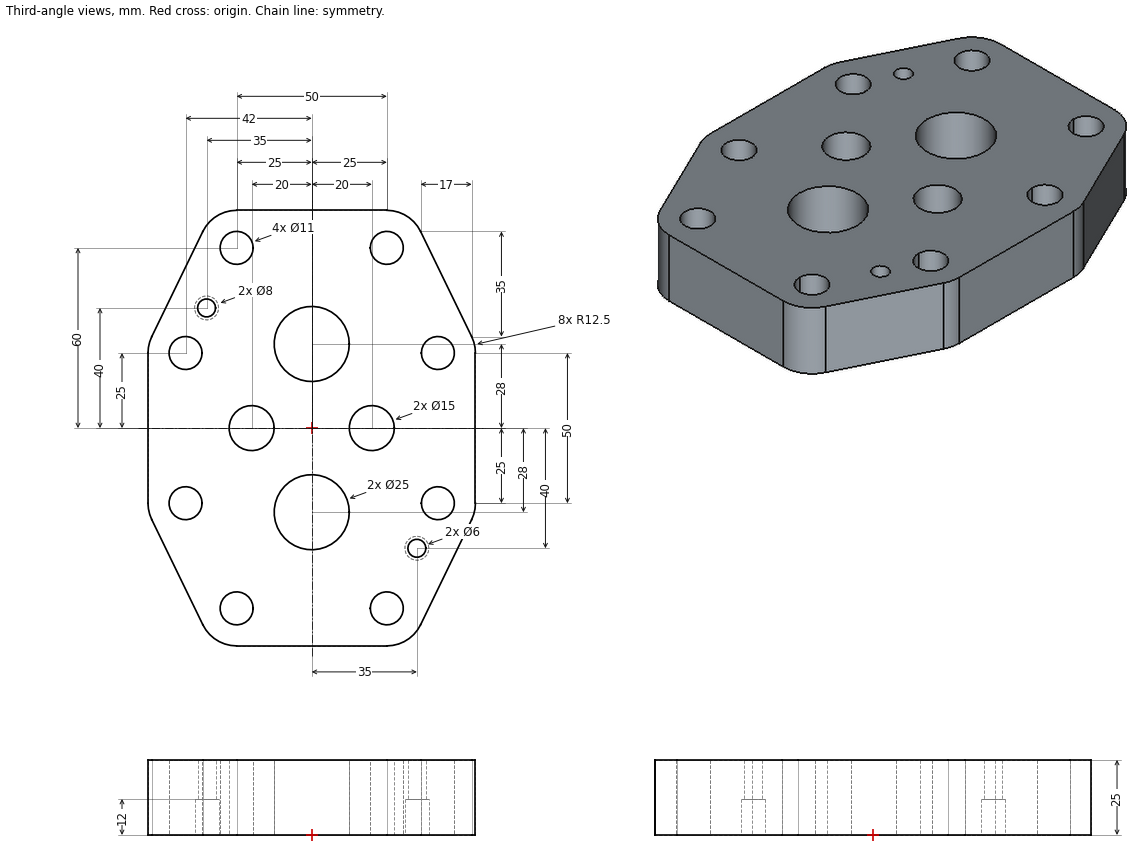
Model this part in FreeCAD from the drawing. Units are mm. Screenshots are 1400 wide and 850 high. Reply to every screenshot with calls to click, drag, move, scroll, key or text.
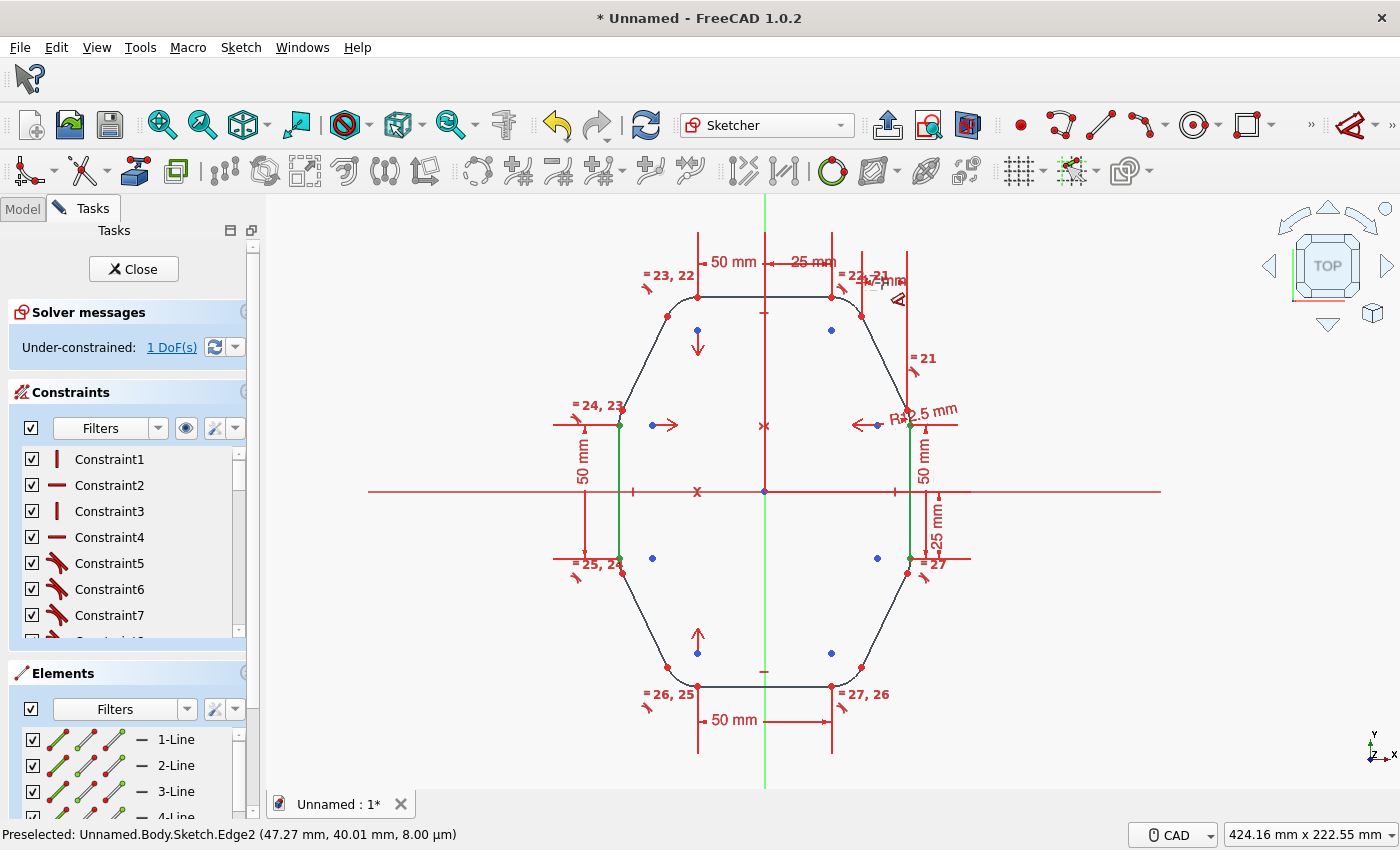
click(894, 382)
click(941, 363)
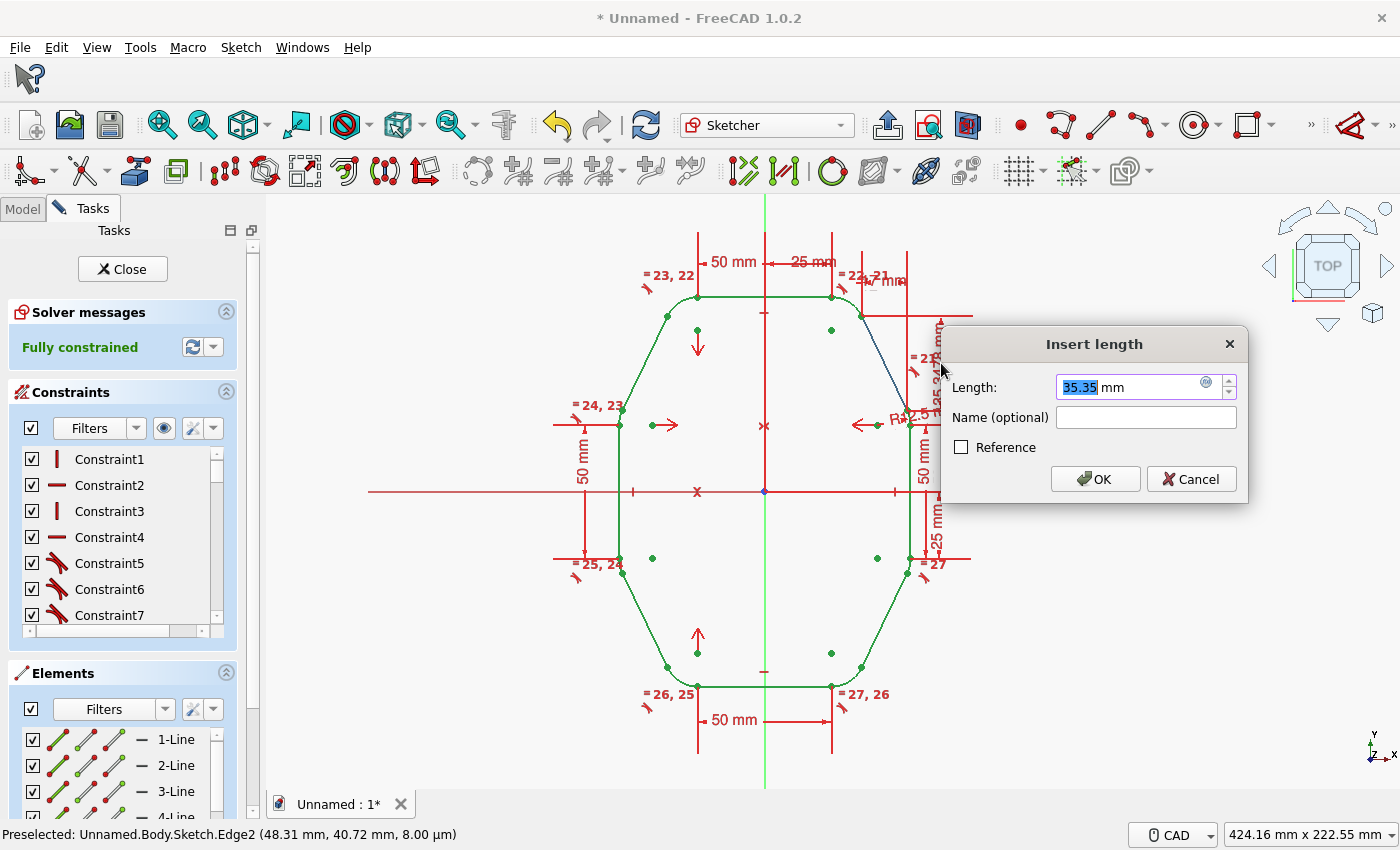
text(35)
key(Return)
key(Escape)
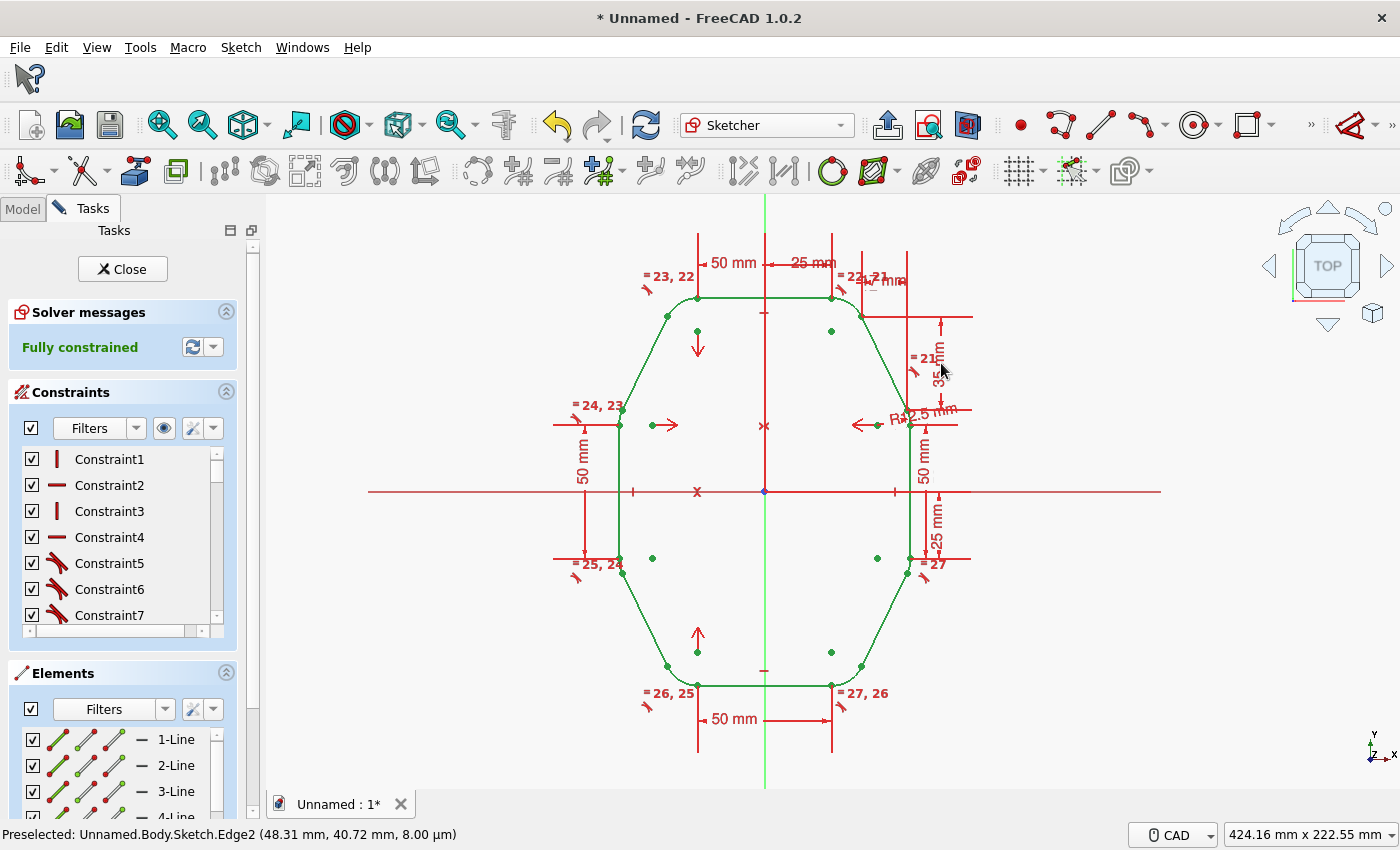
click(123, 269)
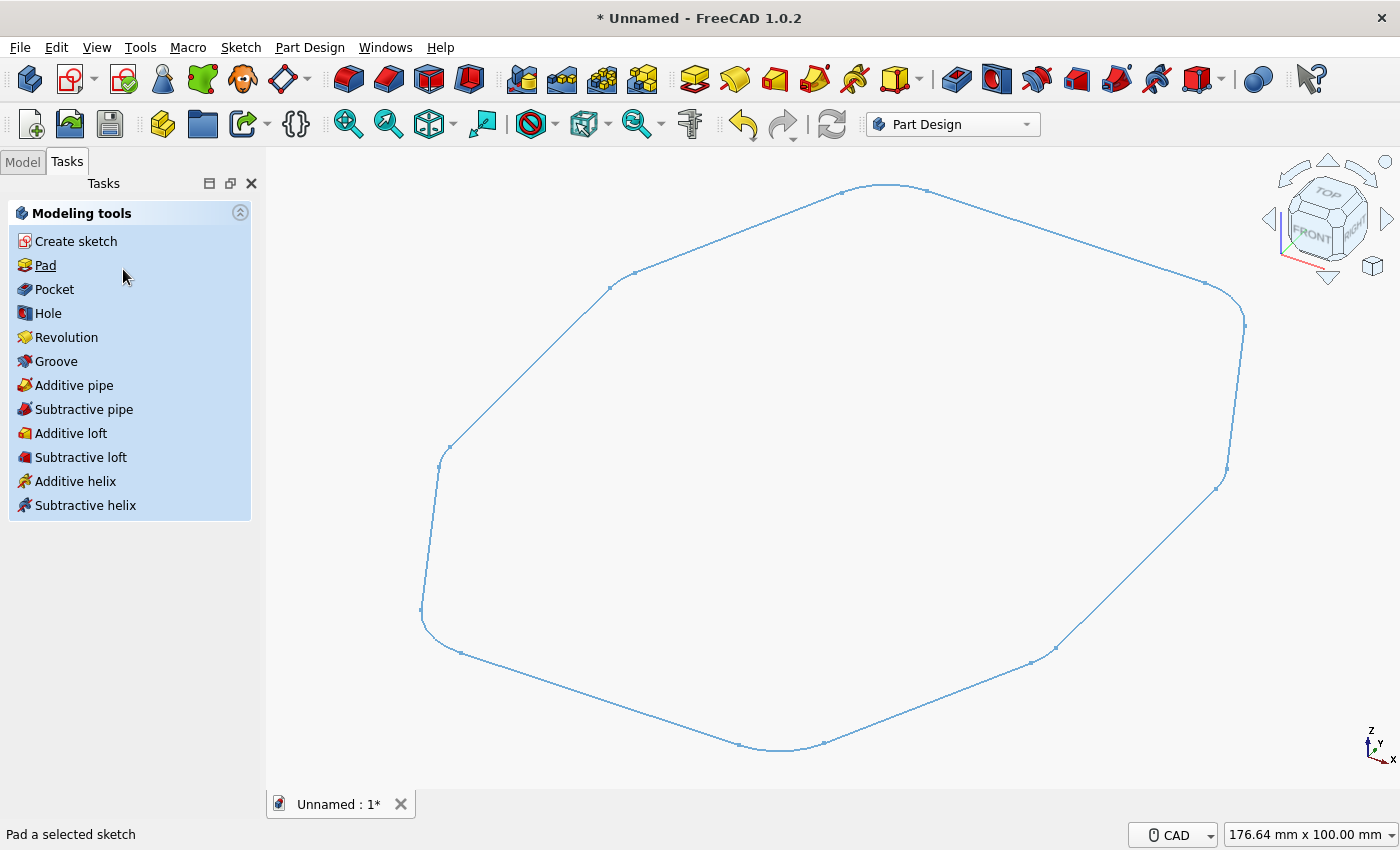
click(696, 80)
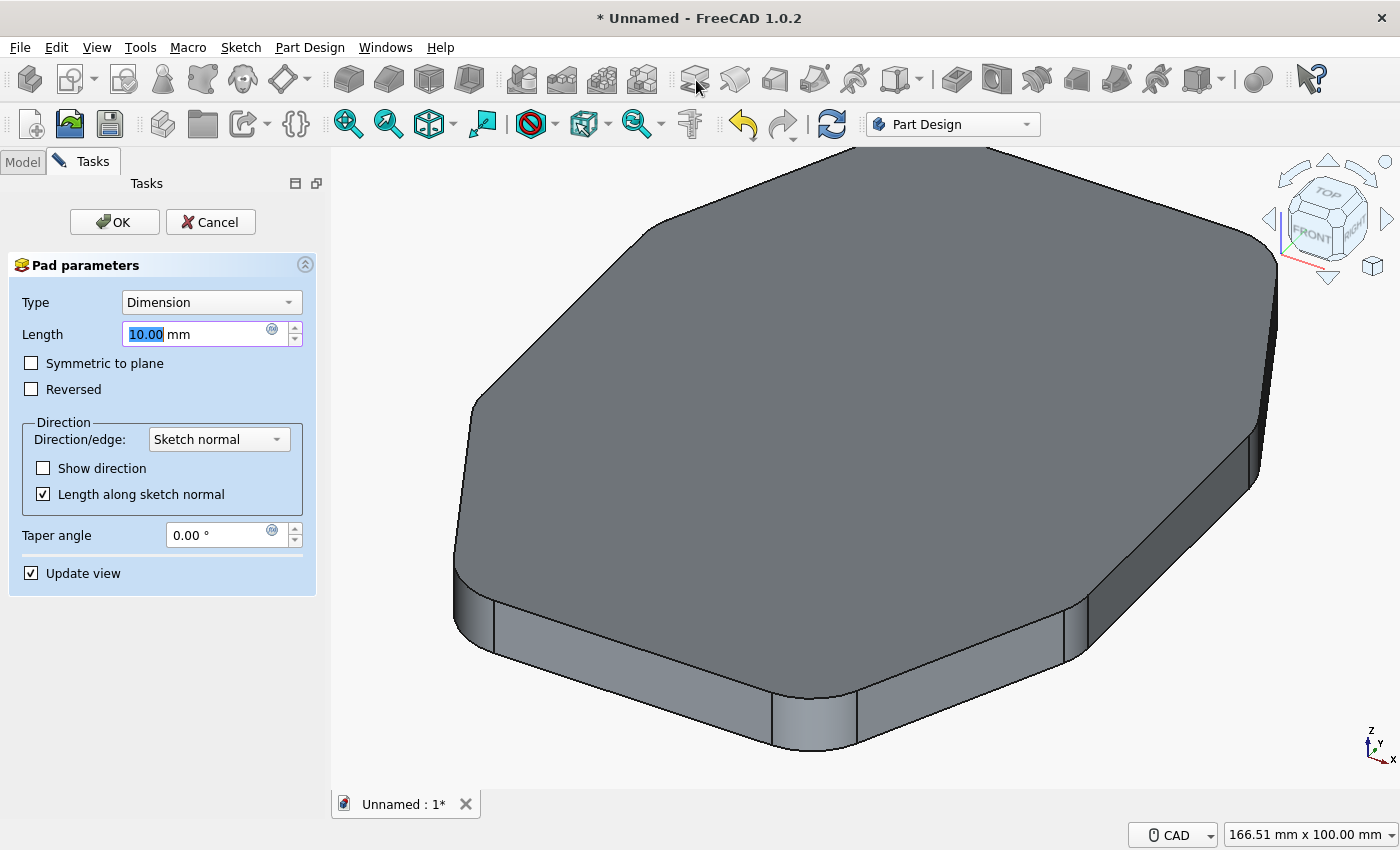
text(25)
key(Tab)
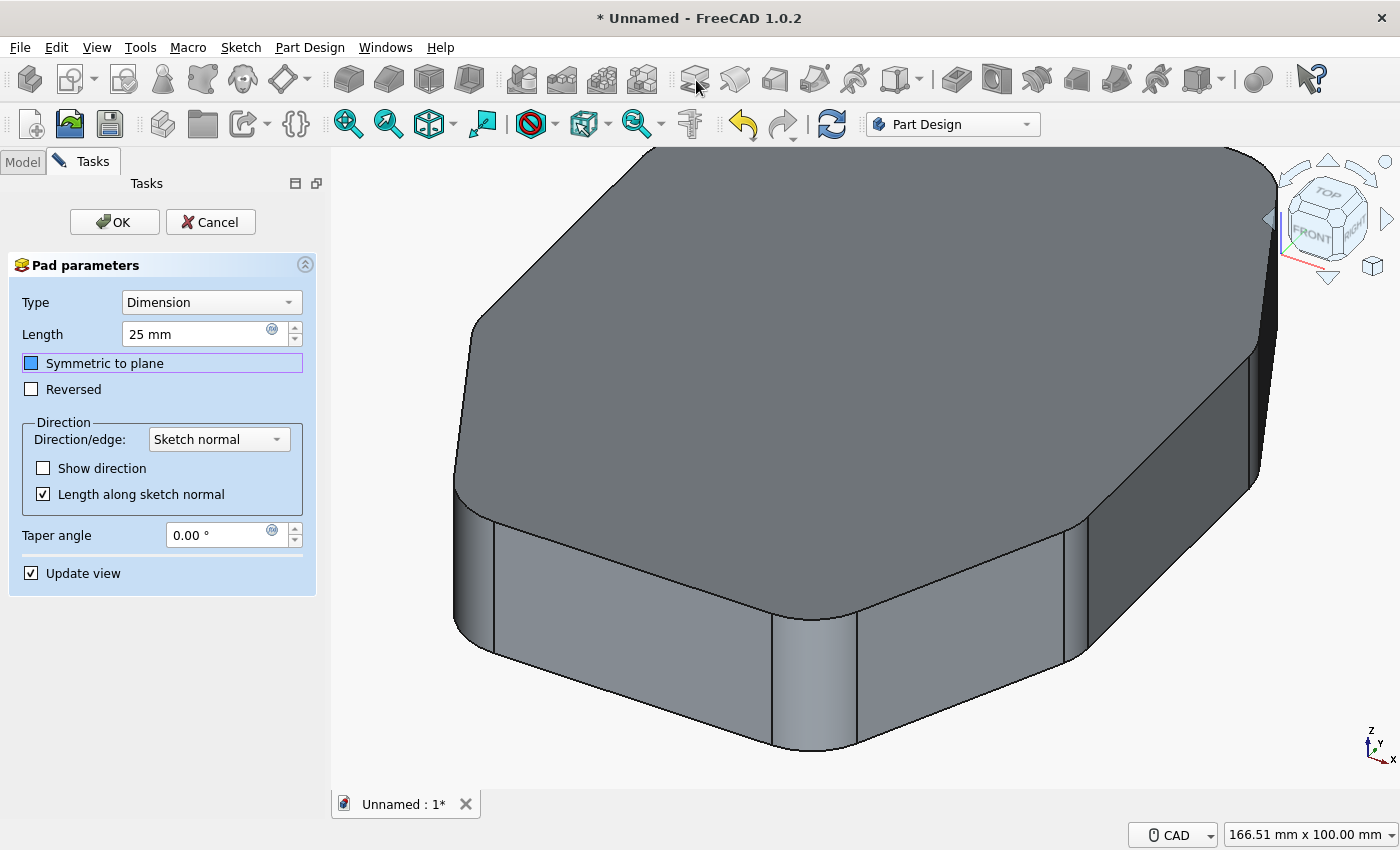
click(115, 222)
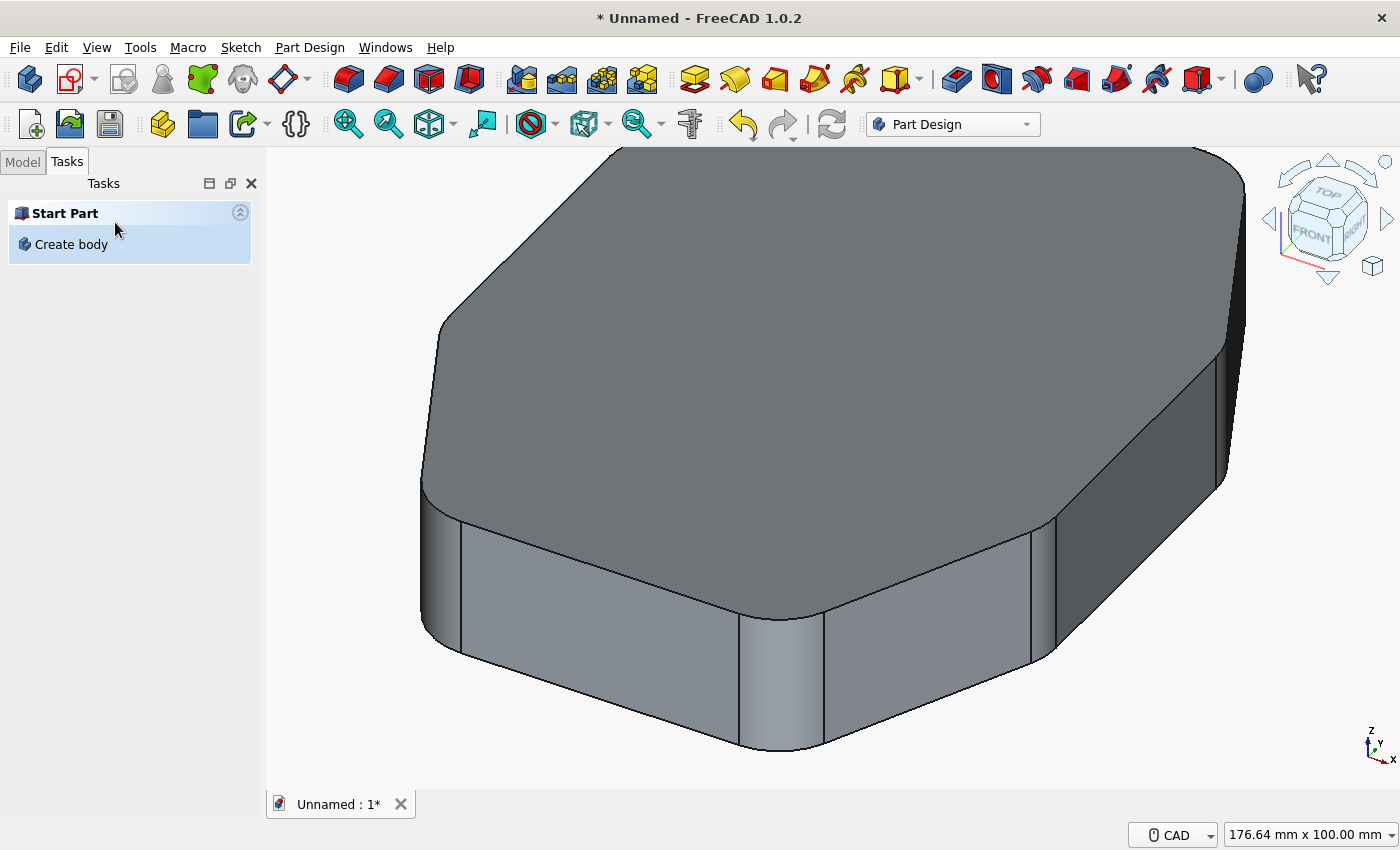
click(350, 124)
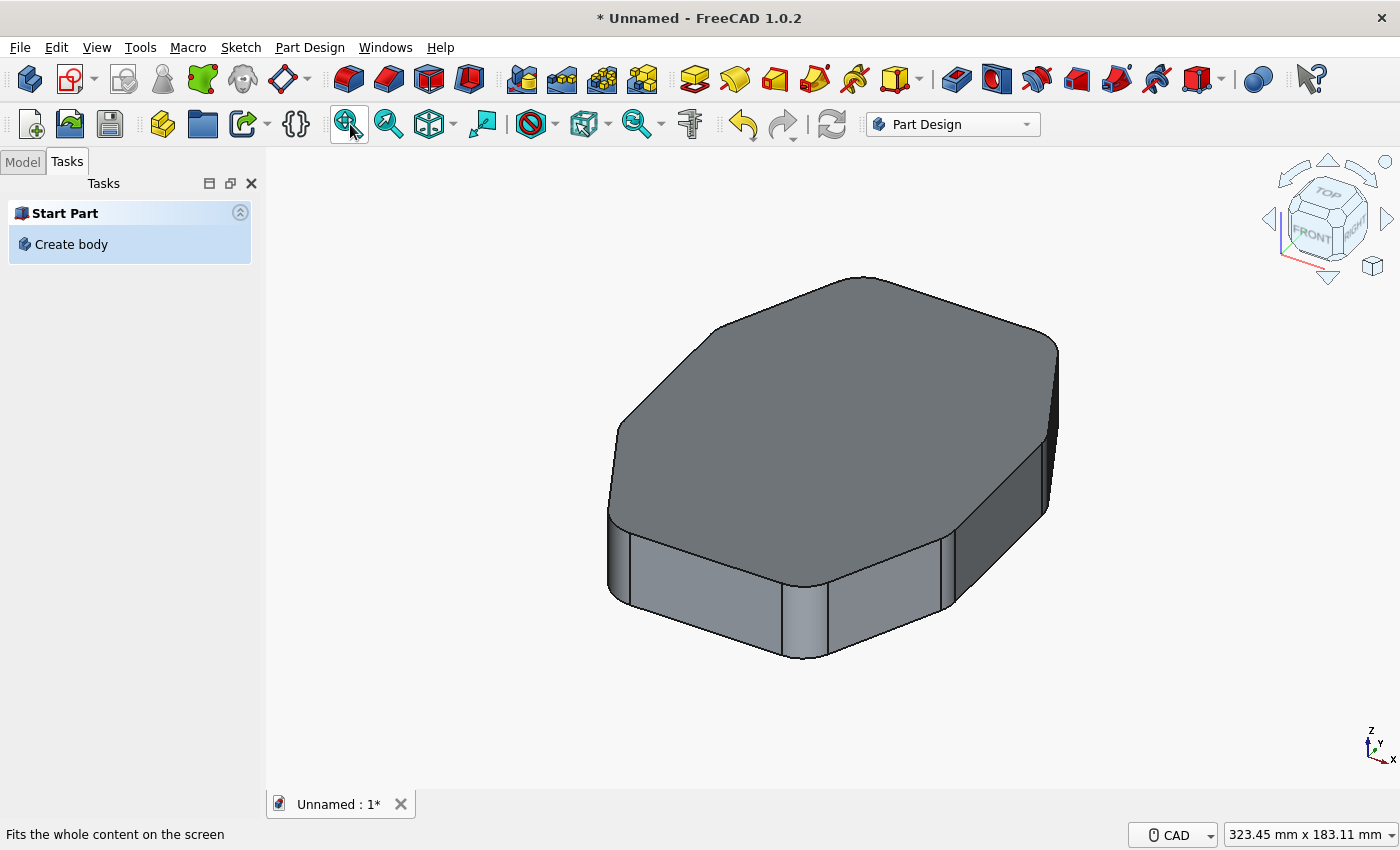
key(5)